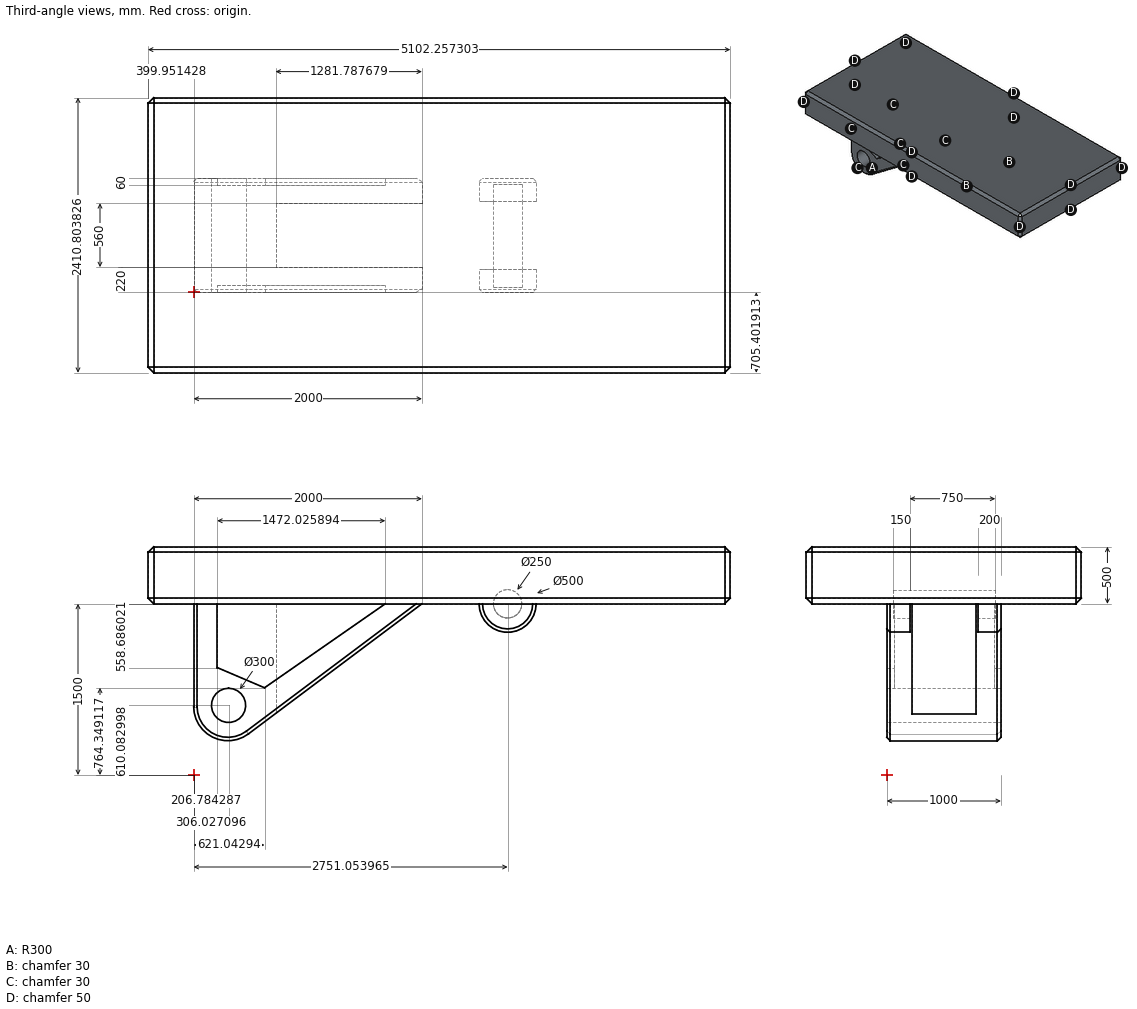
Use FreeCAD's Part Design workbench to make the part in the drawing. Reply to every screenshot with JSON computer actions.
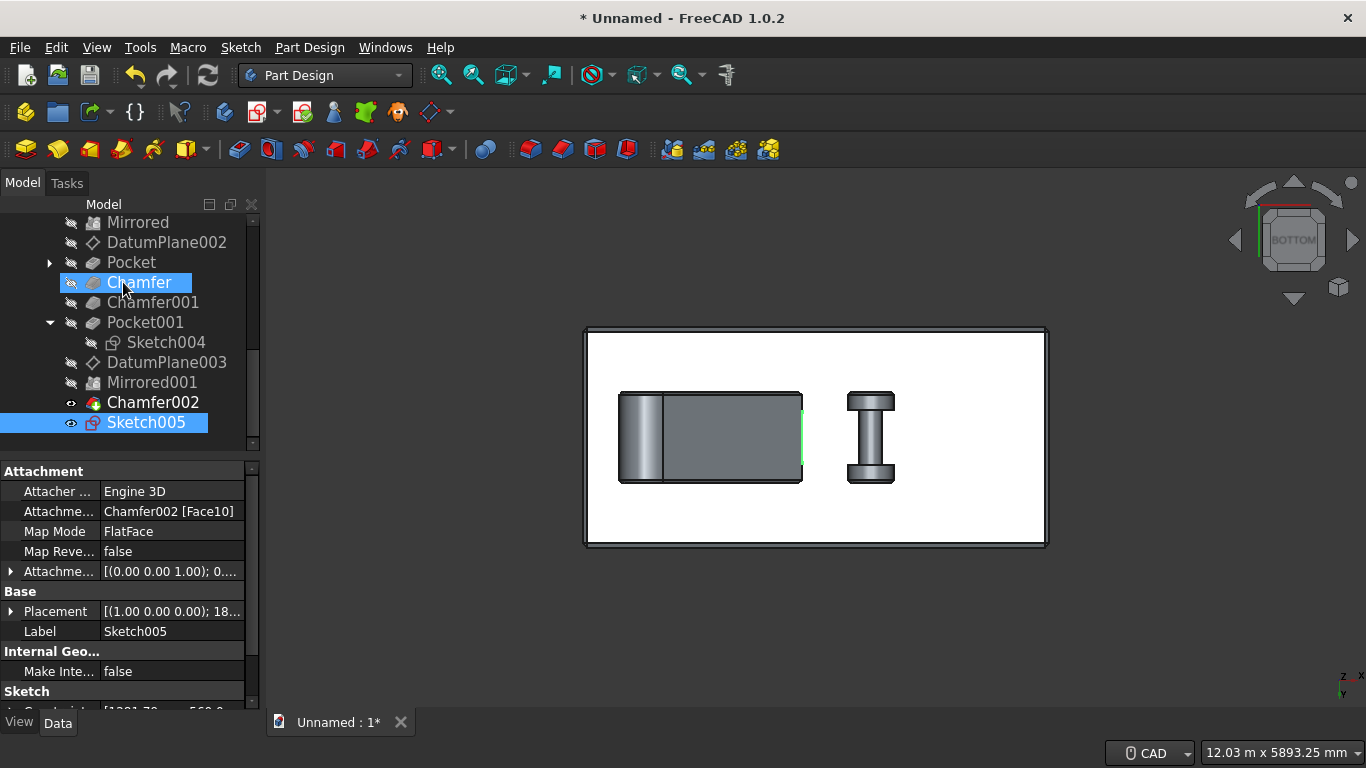
{"action": "left_click", "coordinate": [240, 150]}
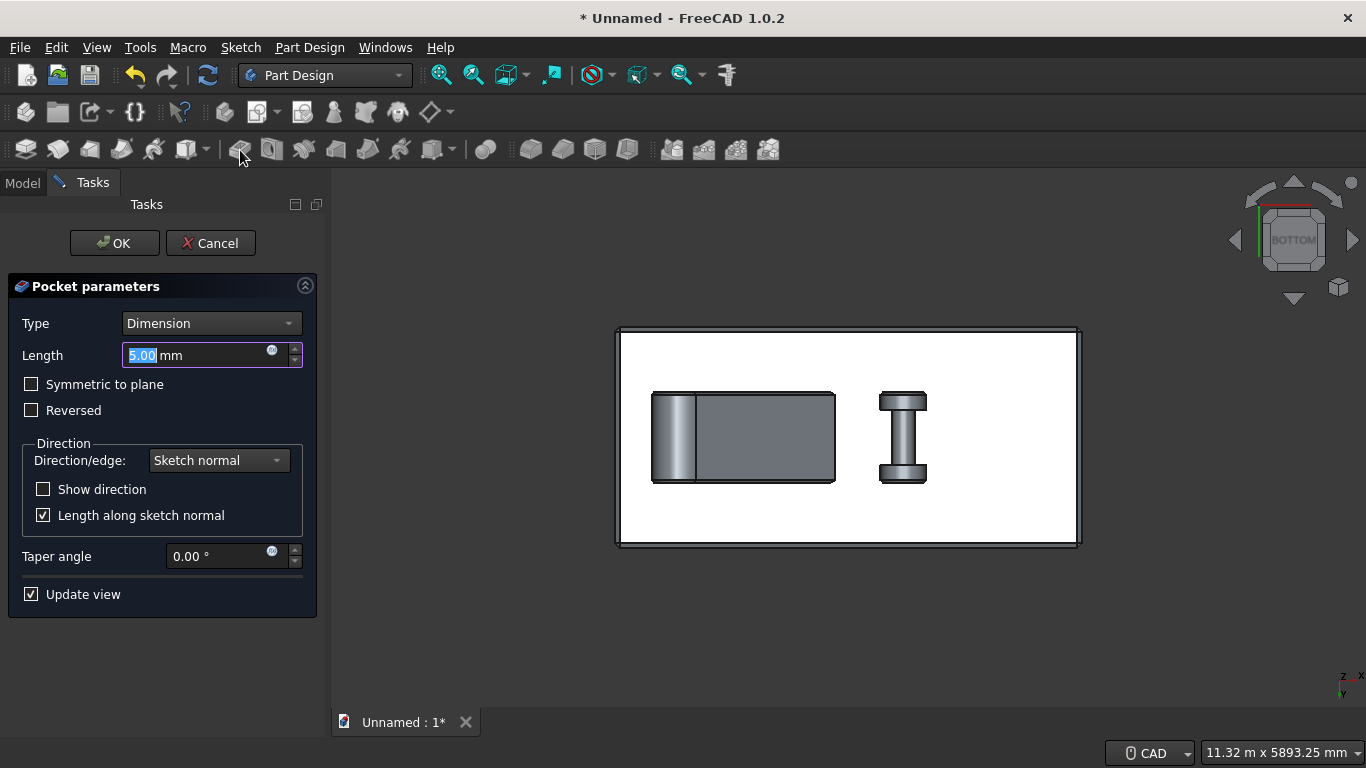
{"action": "left_click", "coordinate": [212, 324]}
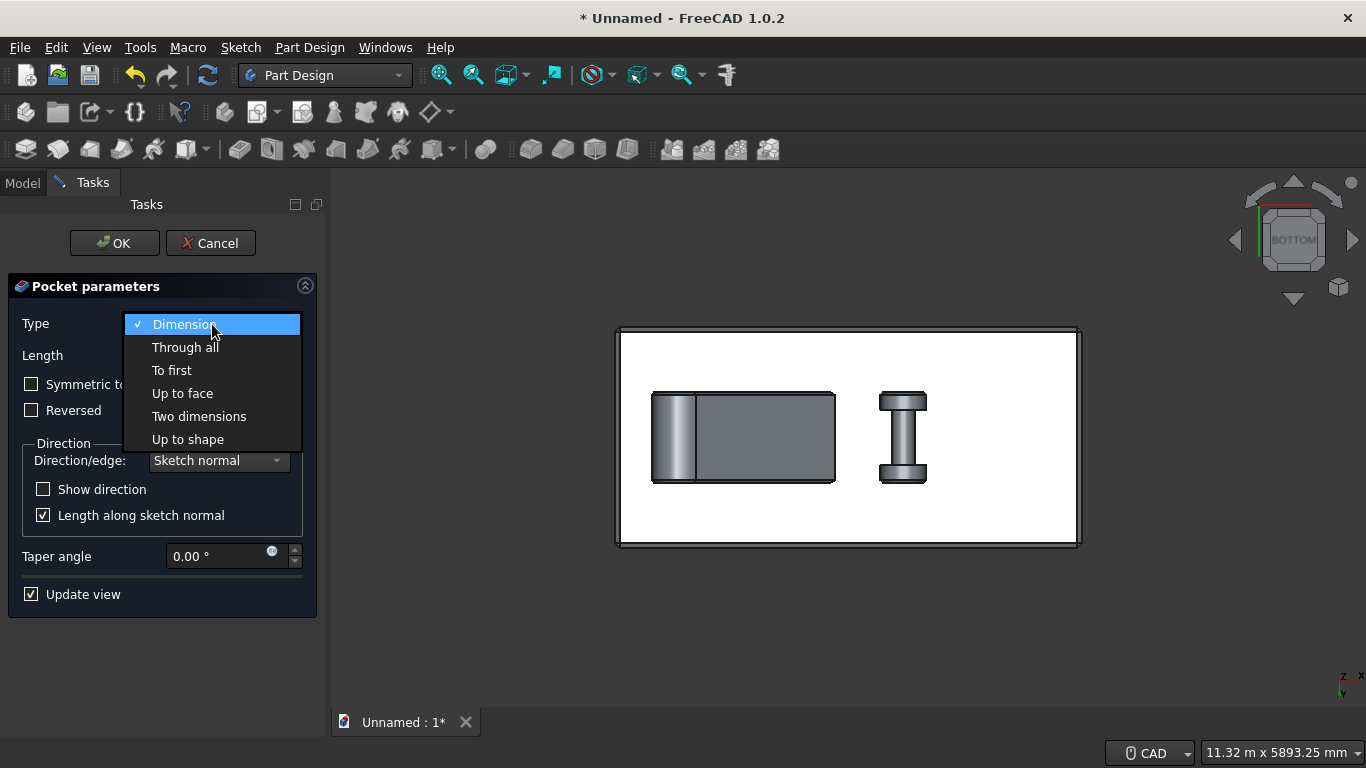
{"action": "left_click", "coordinate": [212, 348]}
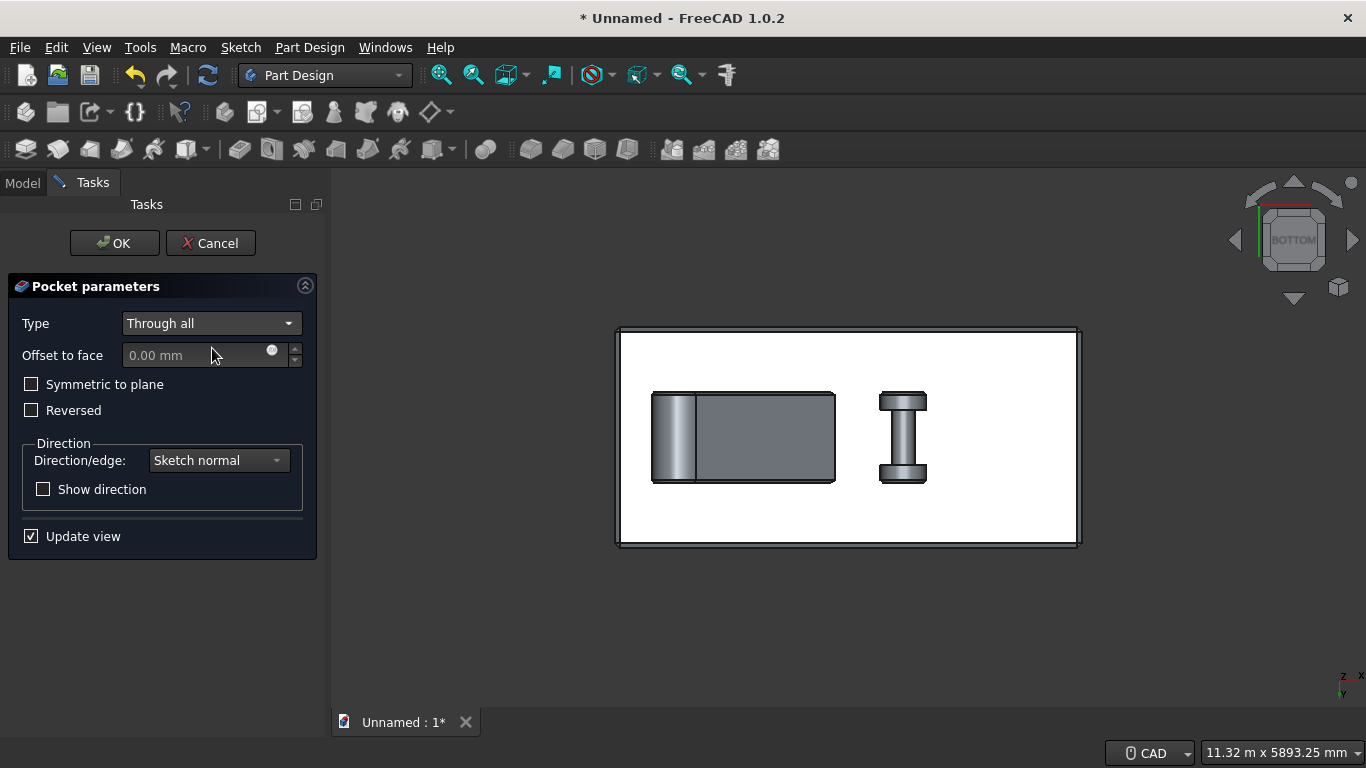
{"action": "left_click", "coordinate": [30, 410]}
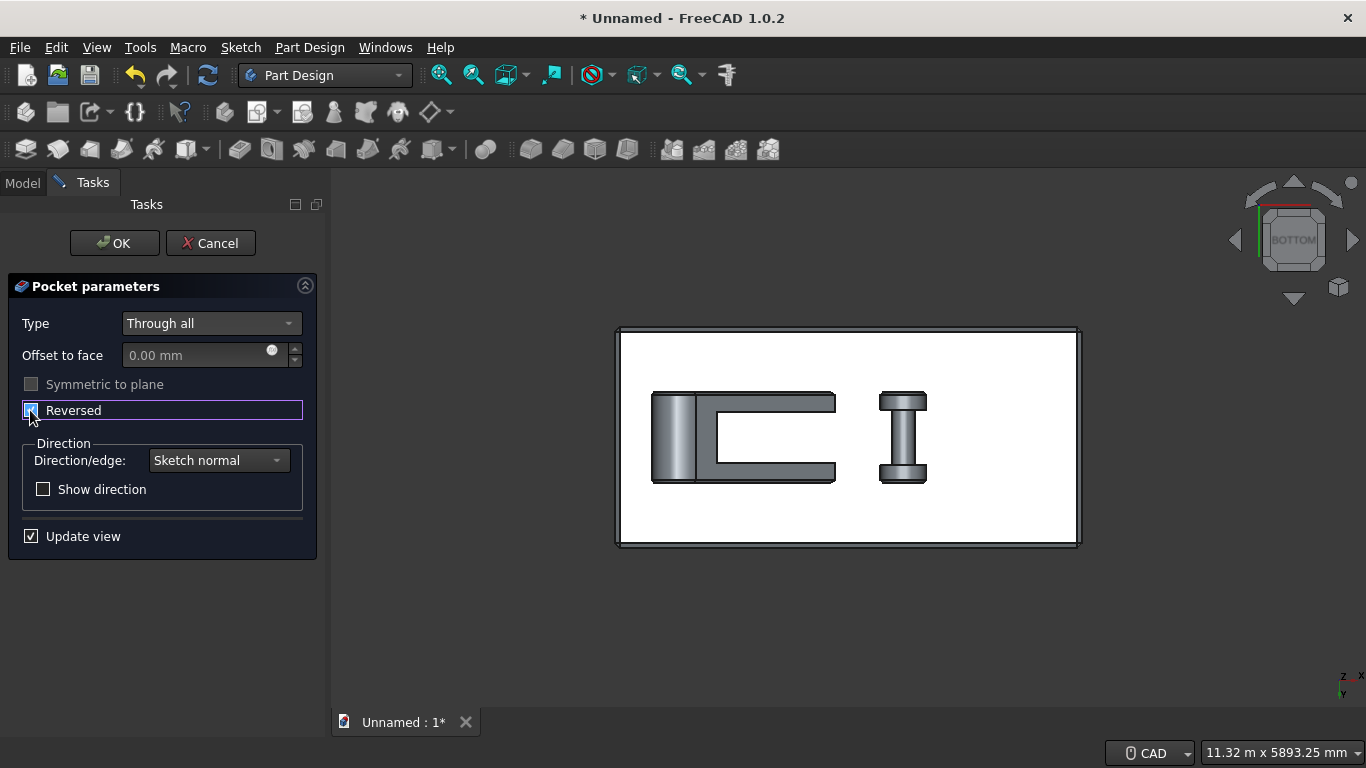
{"action": "left_click", "coordinate": [115, 243]}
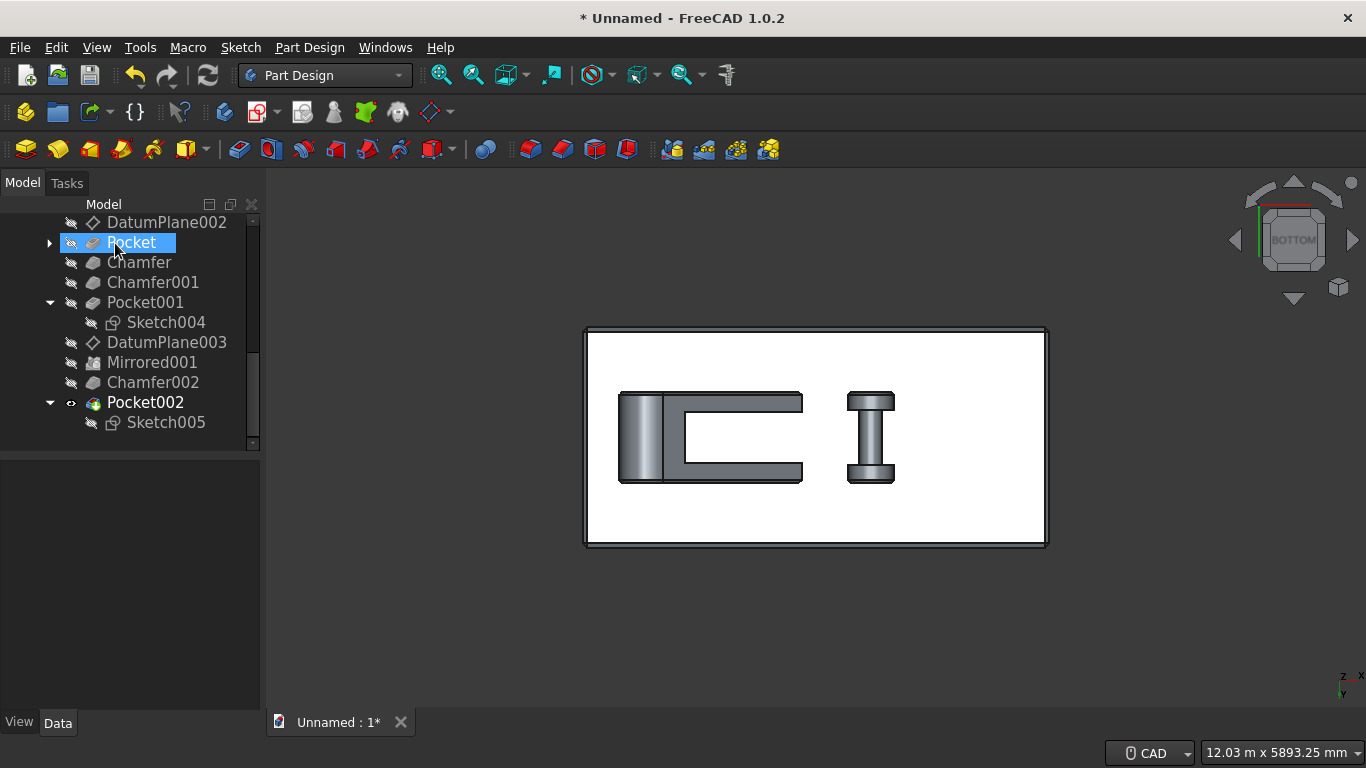
{"action": "key", "text": "0"}